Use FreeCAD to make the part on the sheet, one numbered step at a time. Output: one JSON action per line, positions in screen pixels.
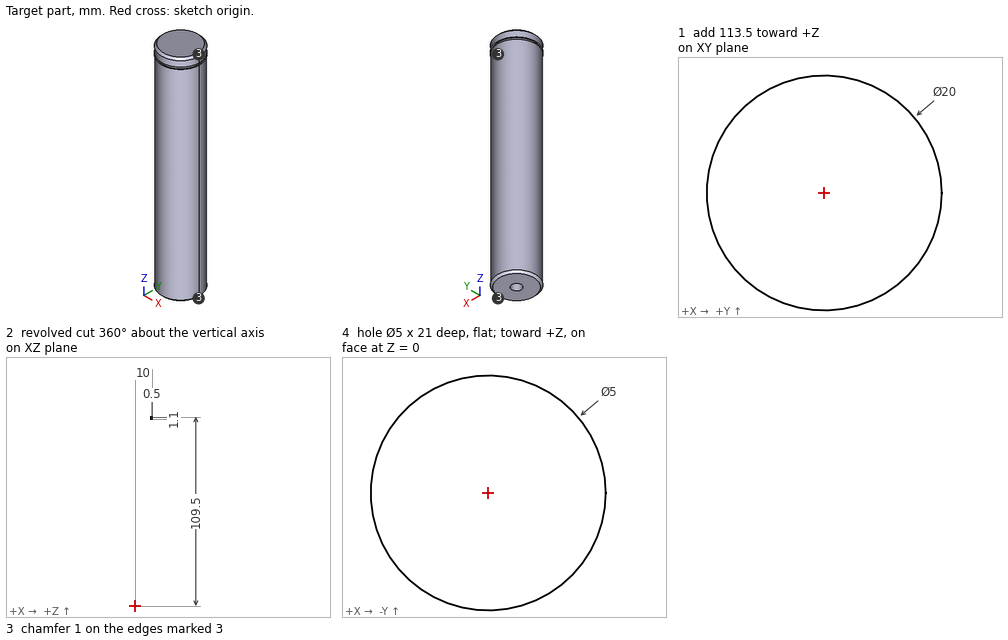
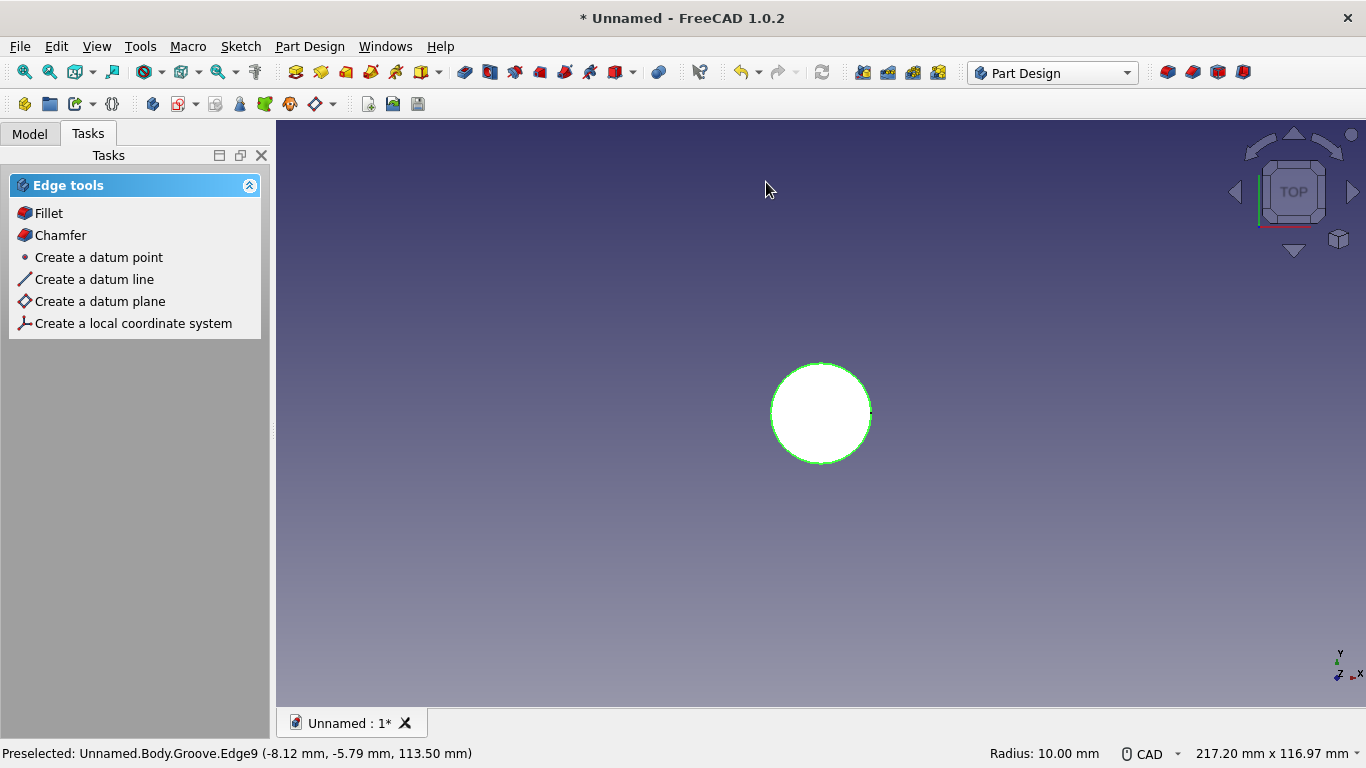
{"action": "key", "text": "v f"}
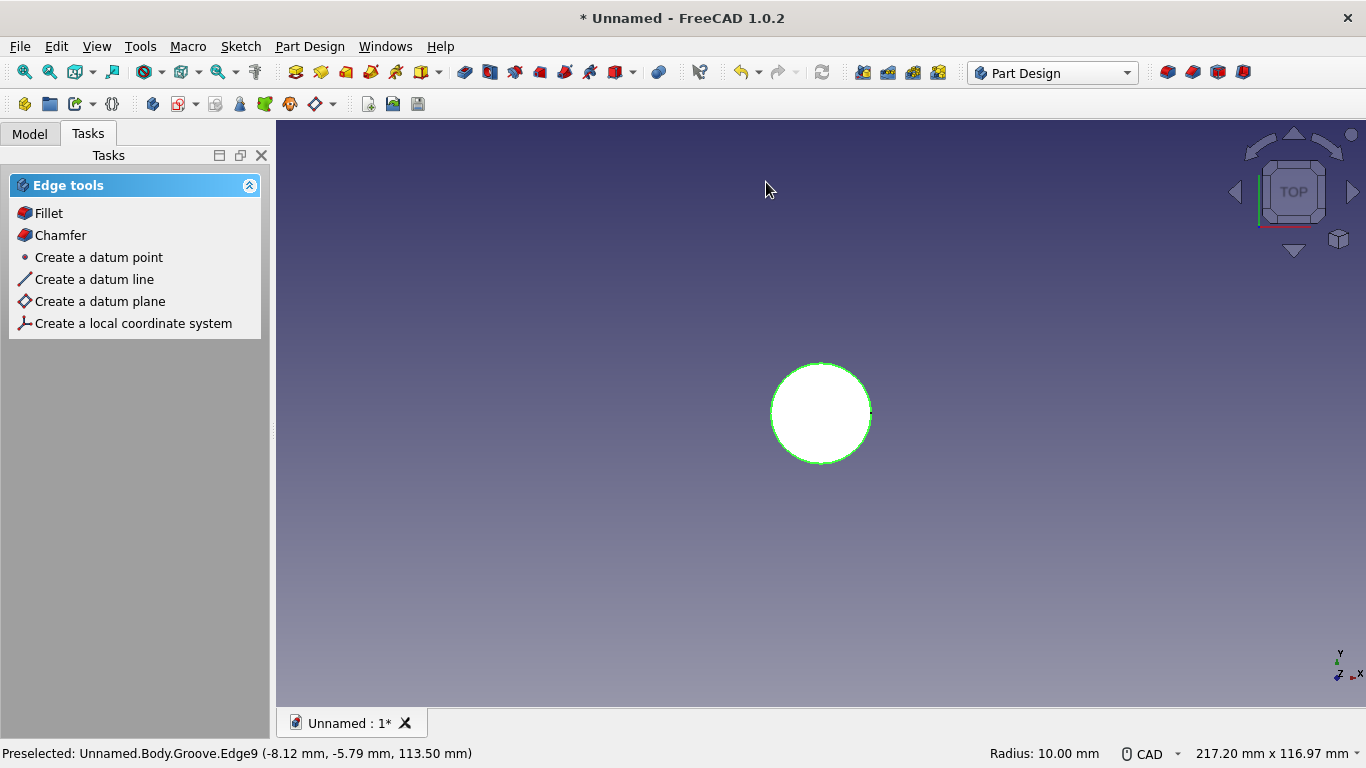
{"action": "key", "text": "1"}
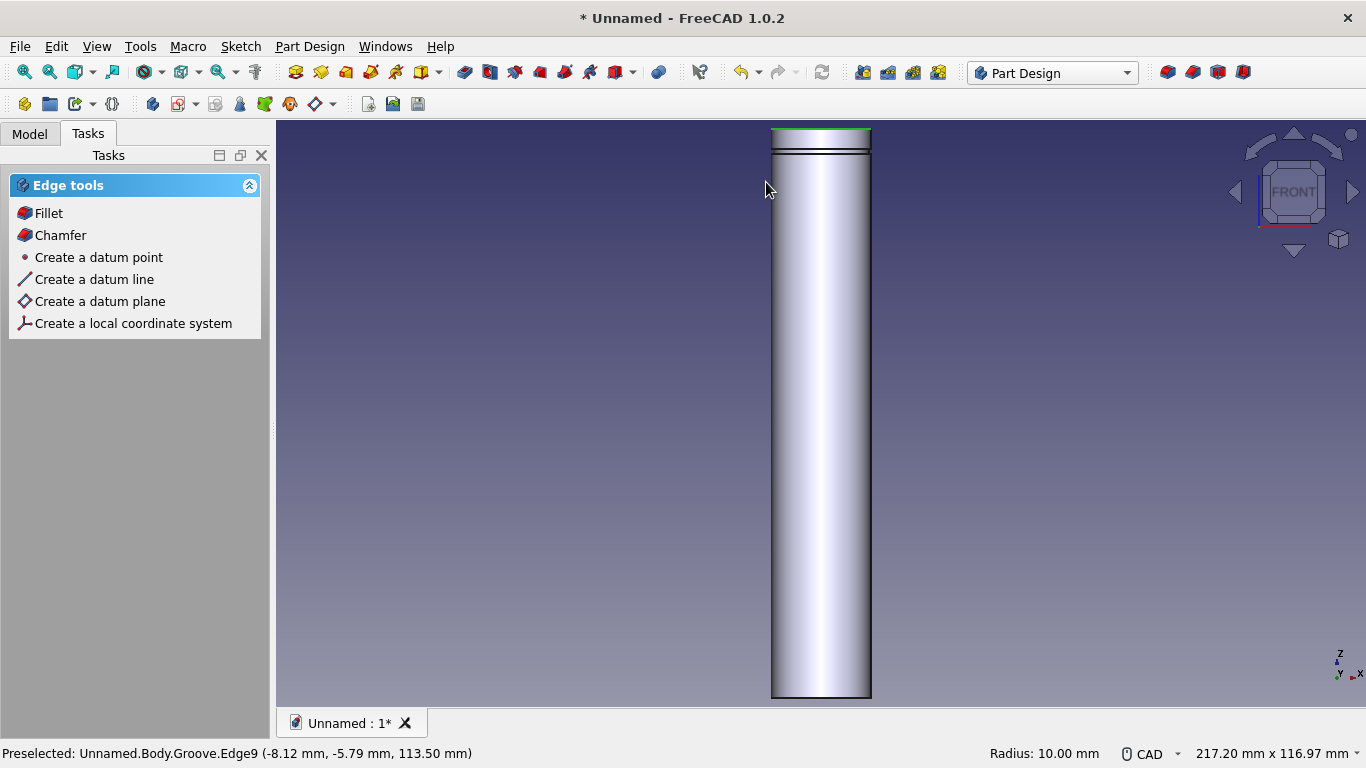
{"action": "key", "text": "3"}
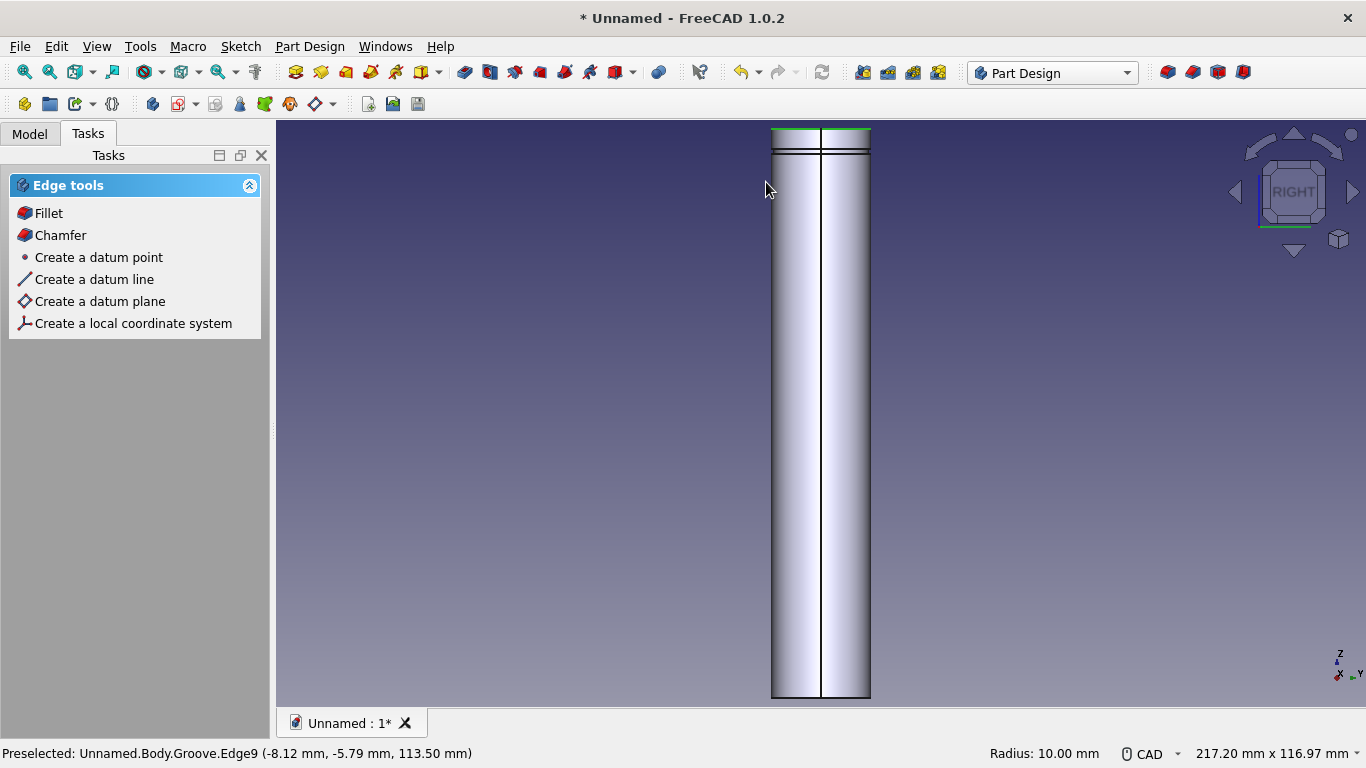
{"action": "key", "text": "5"}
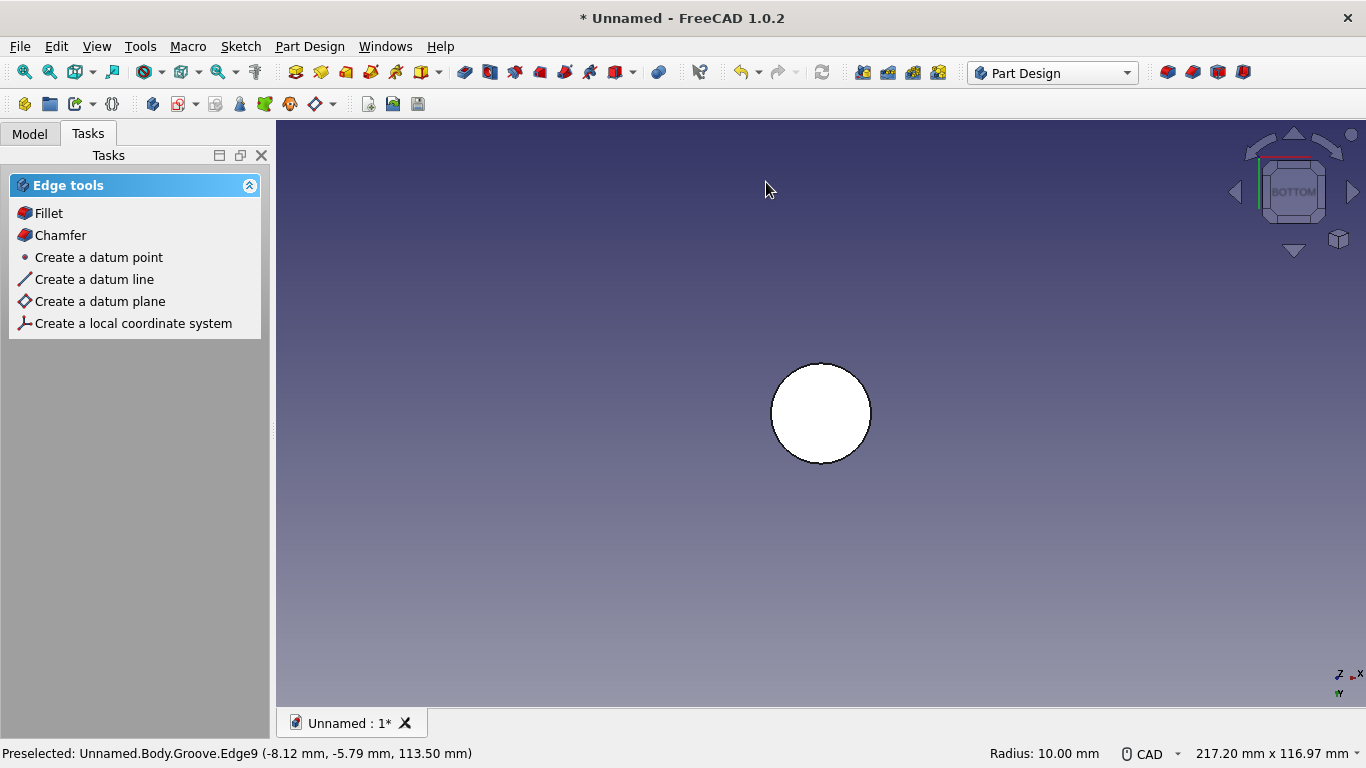
{"action": "key", "text": "v f"}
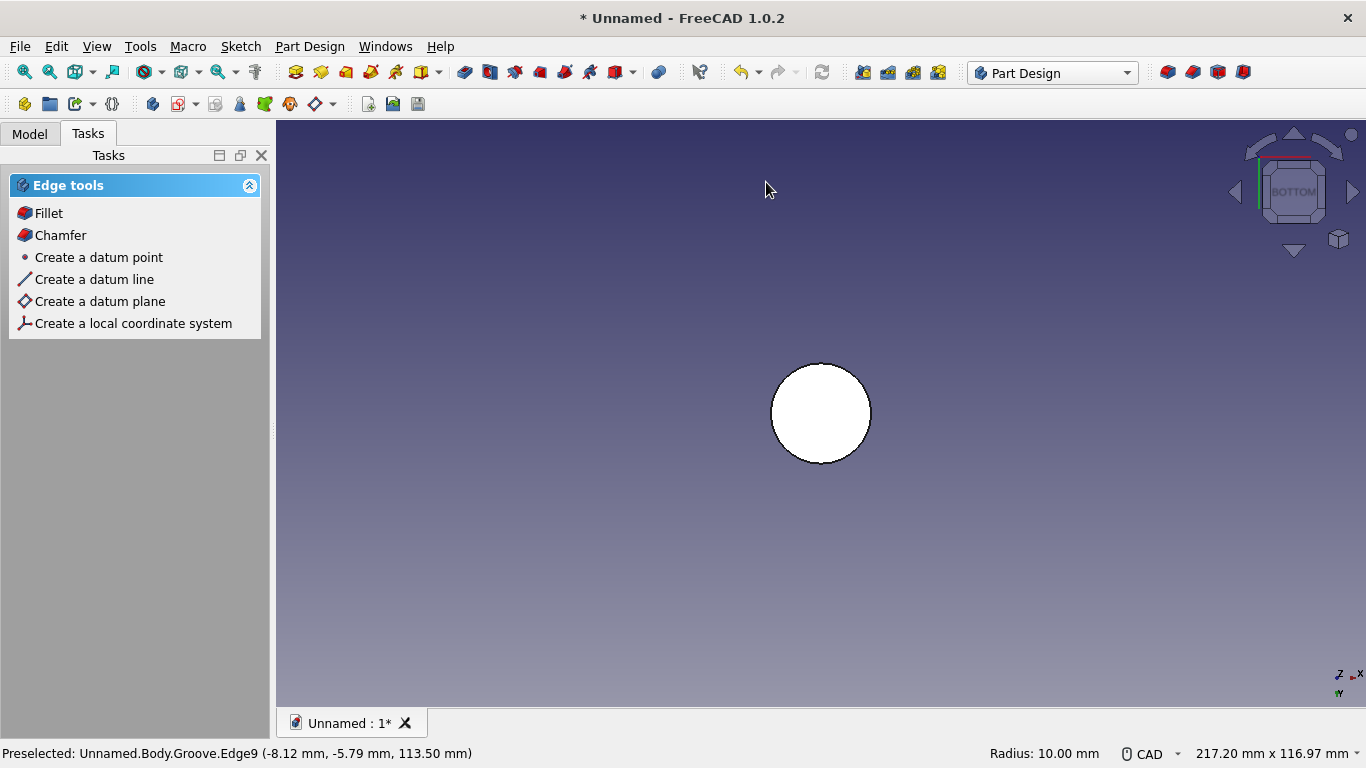
{"action": "left_click", "coordinate": [771, 412], "text": "ctrl"}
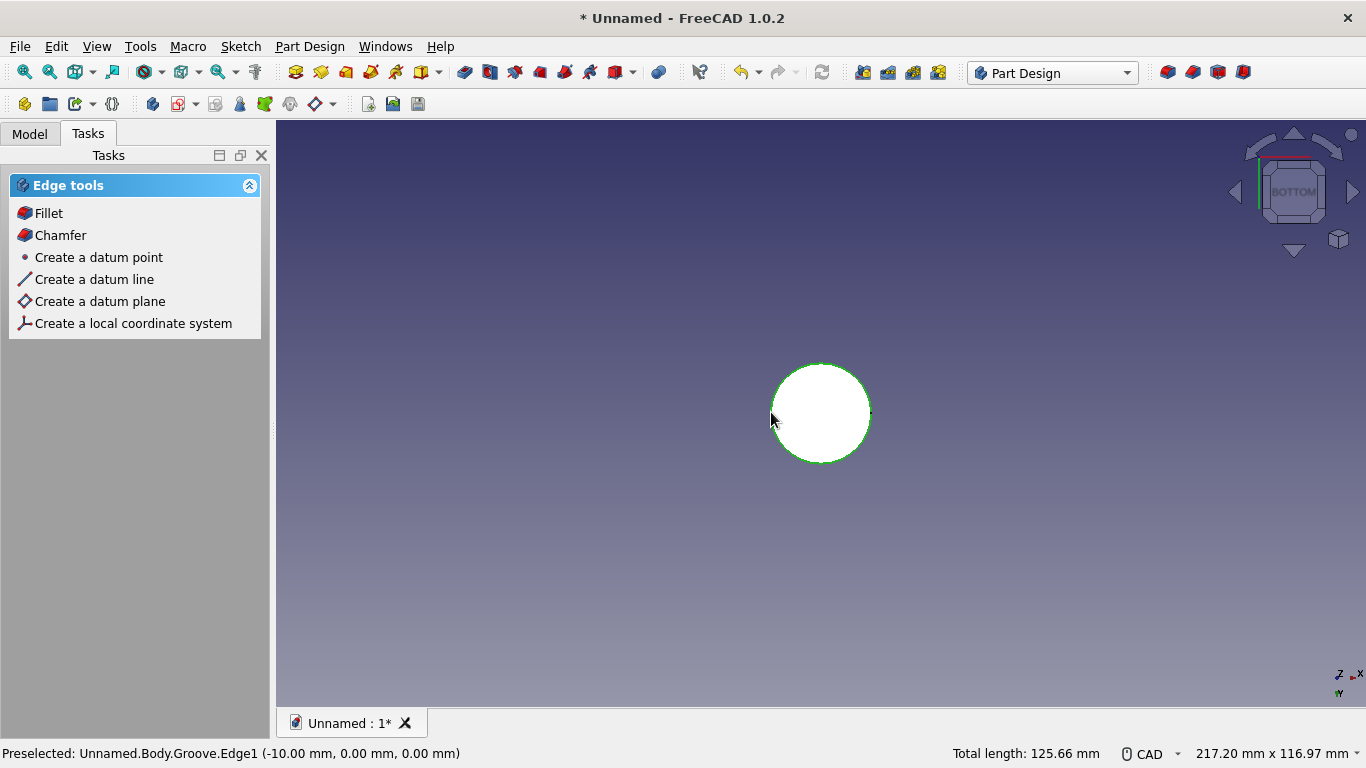
{"action": "left_click", "coordinate": [1193, 72]}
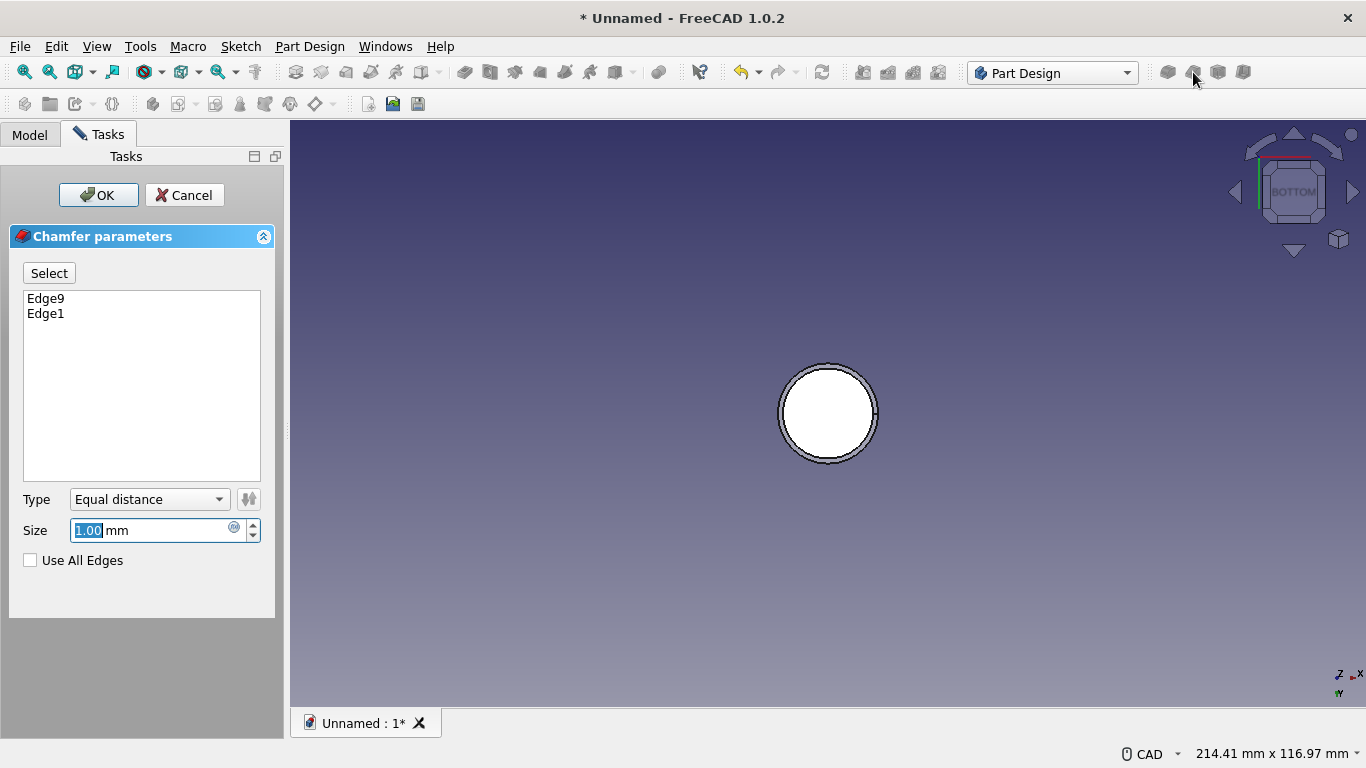
{"action": "type", "text": "1"}
{"action": "key", "text": "Tab"}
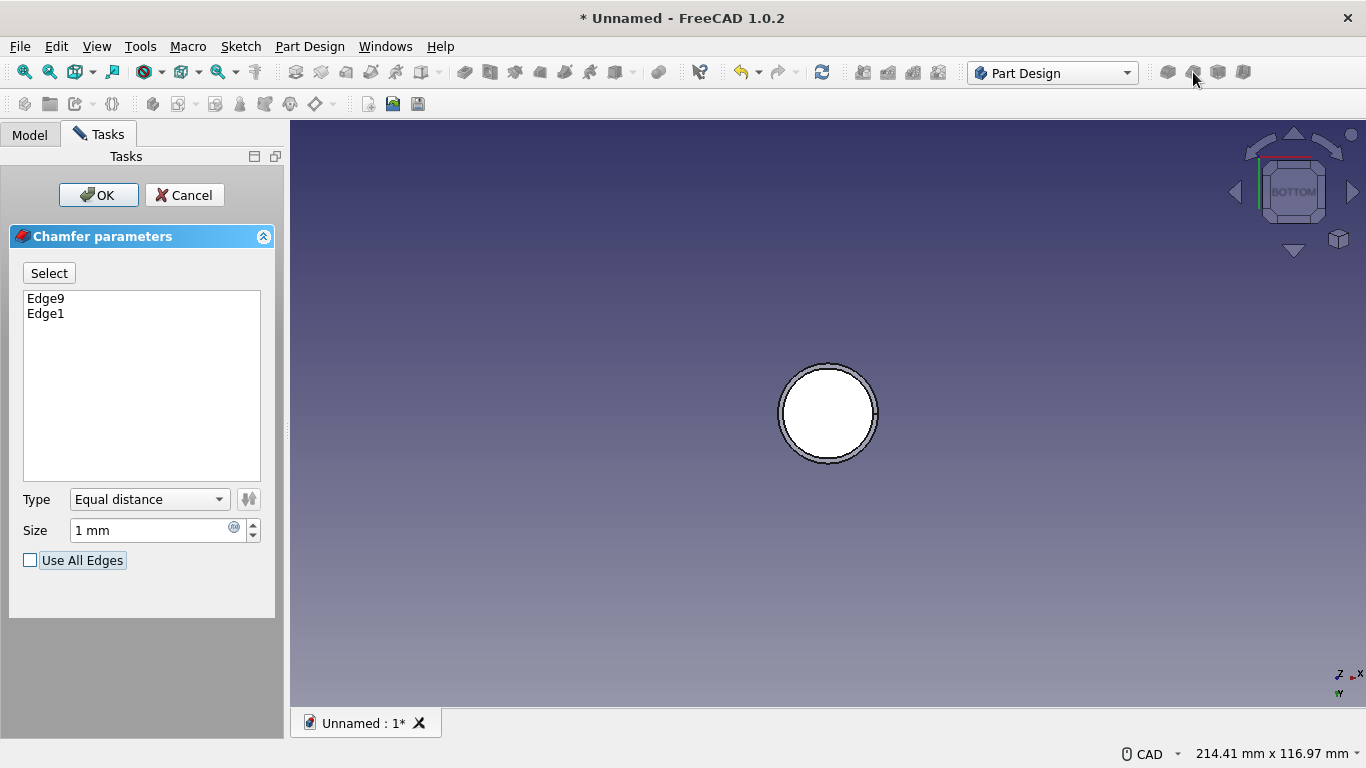
{"action": "left_click", "coordinate": [99, 195]}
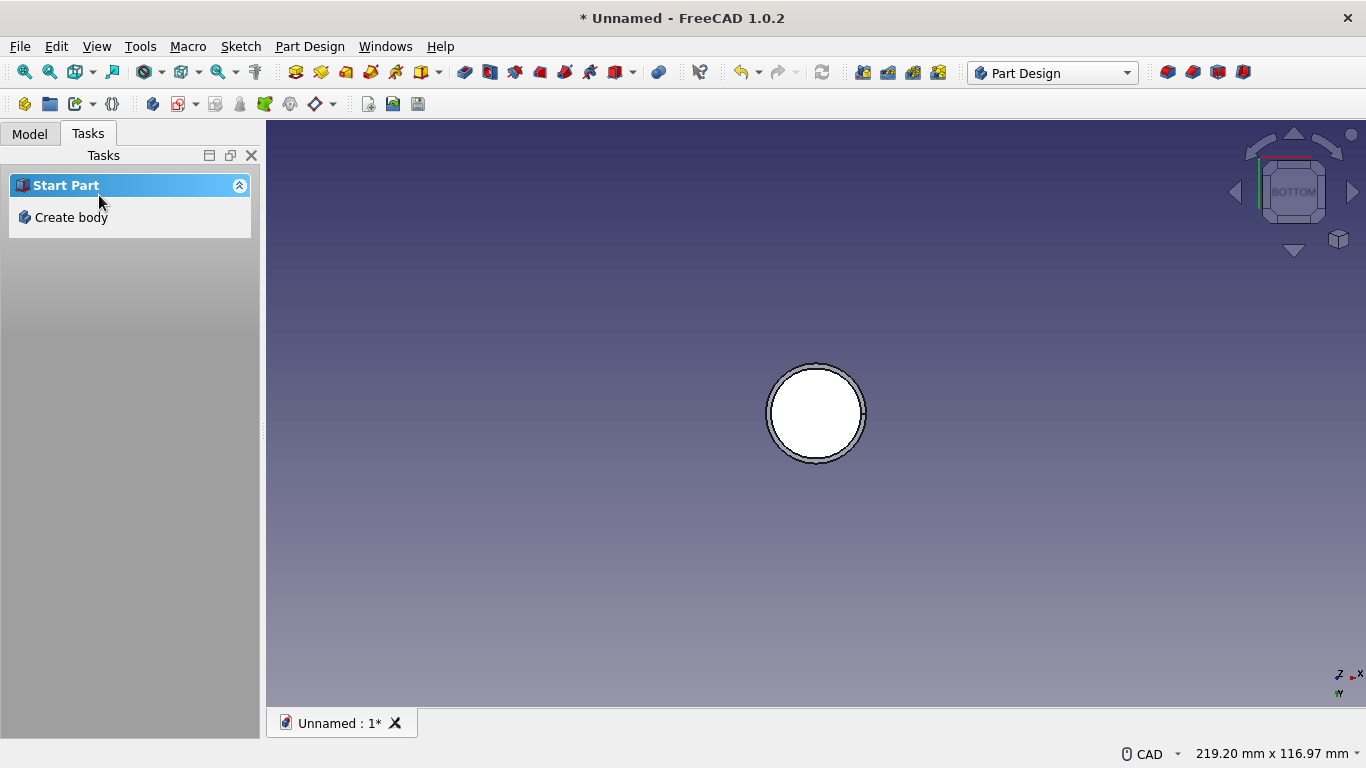
{"action": "key", "text": "v f"}